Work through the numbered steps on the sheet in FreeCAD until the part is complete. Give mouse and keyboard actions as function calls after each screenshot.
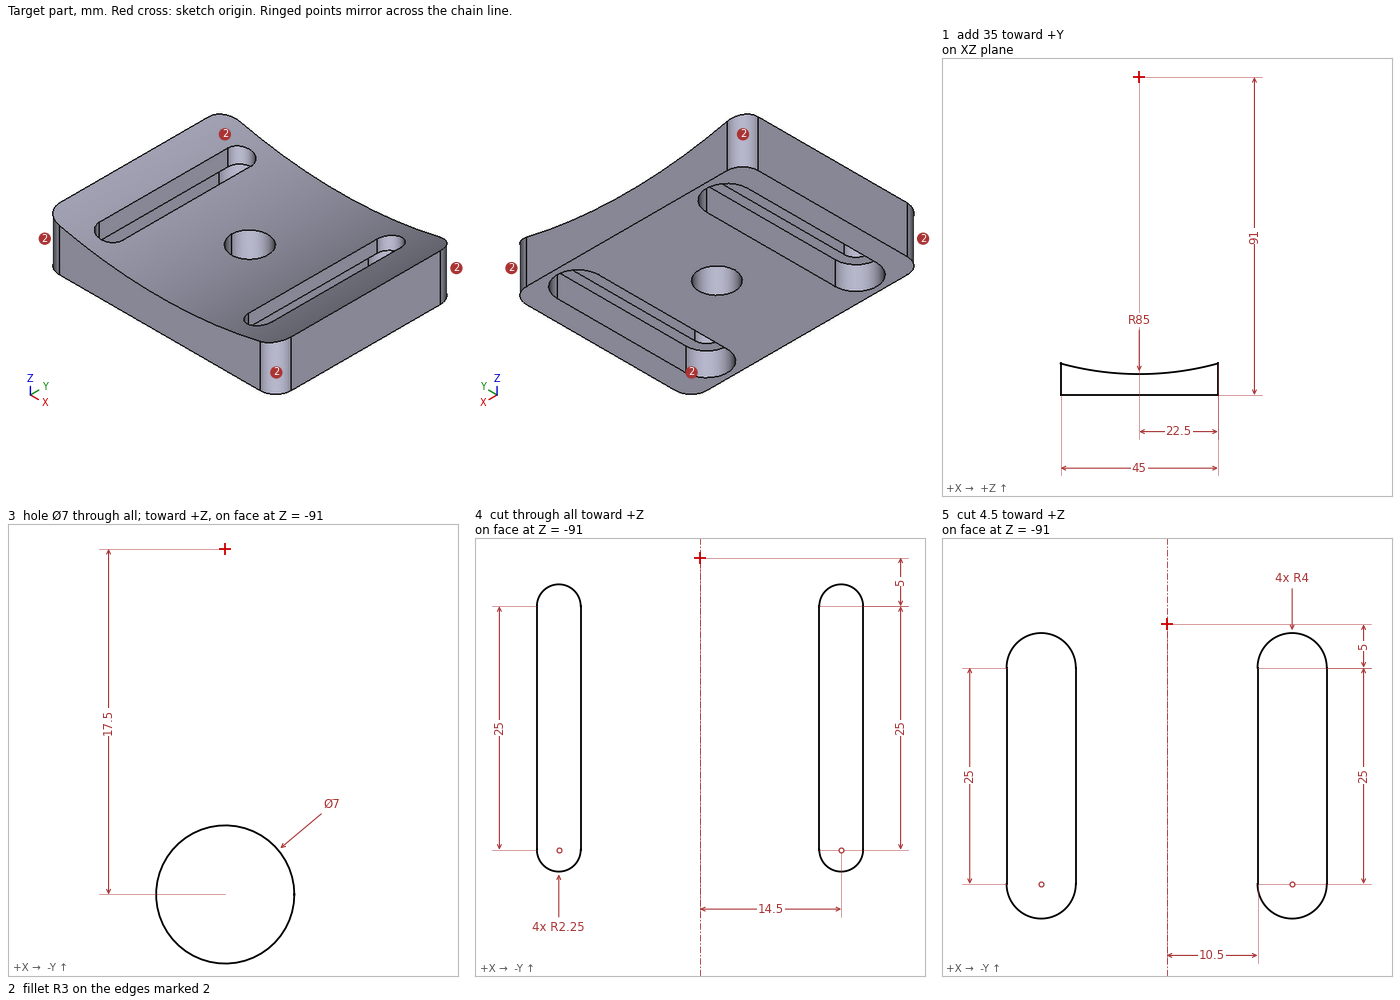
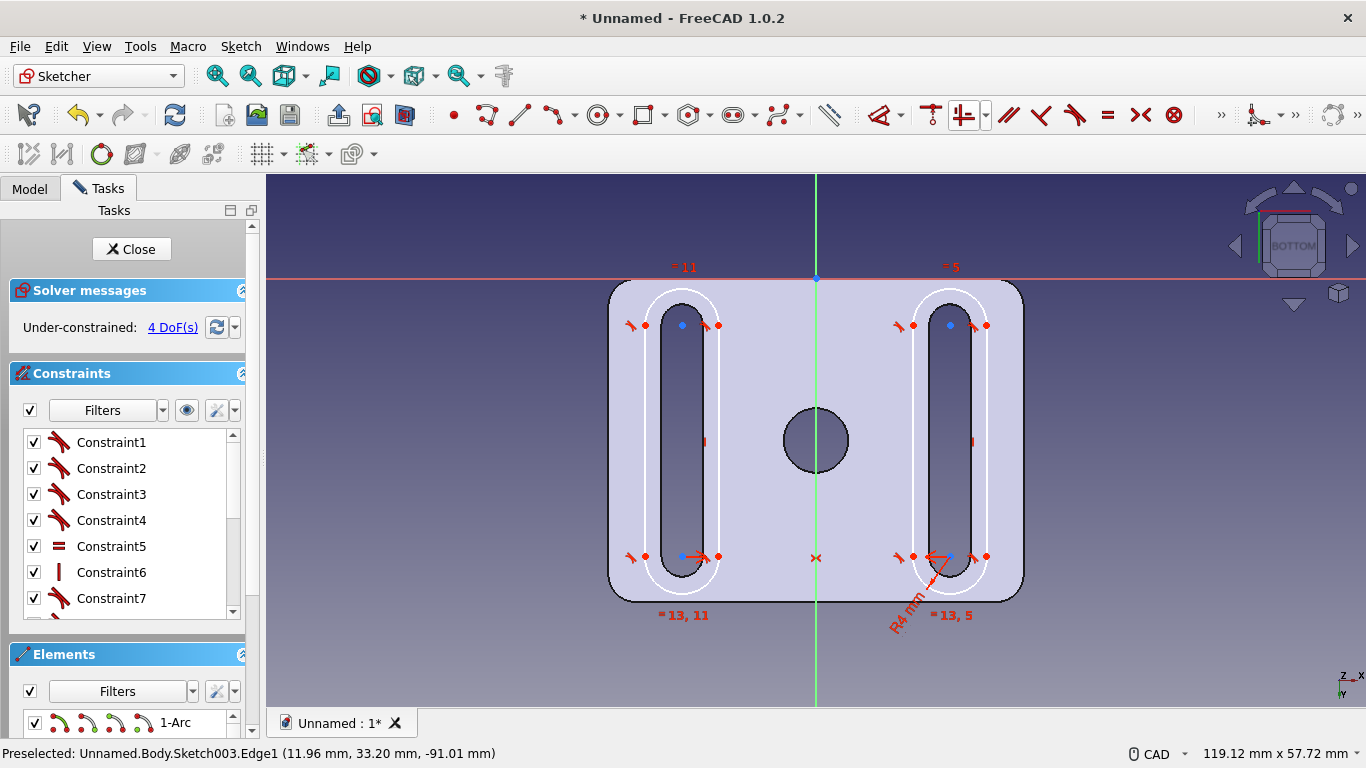
click(913, 488)
click(947, 442)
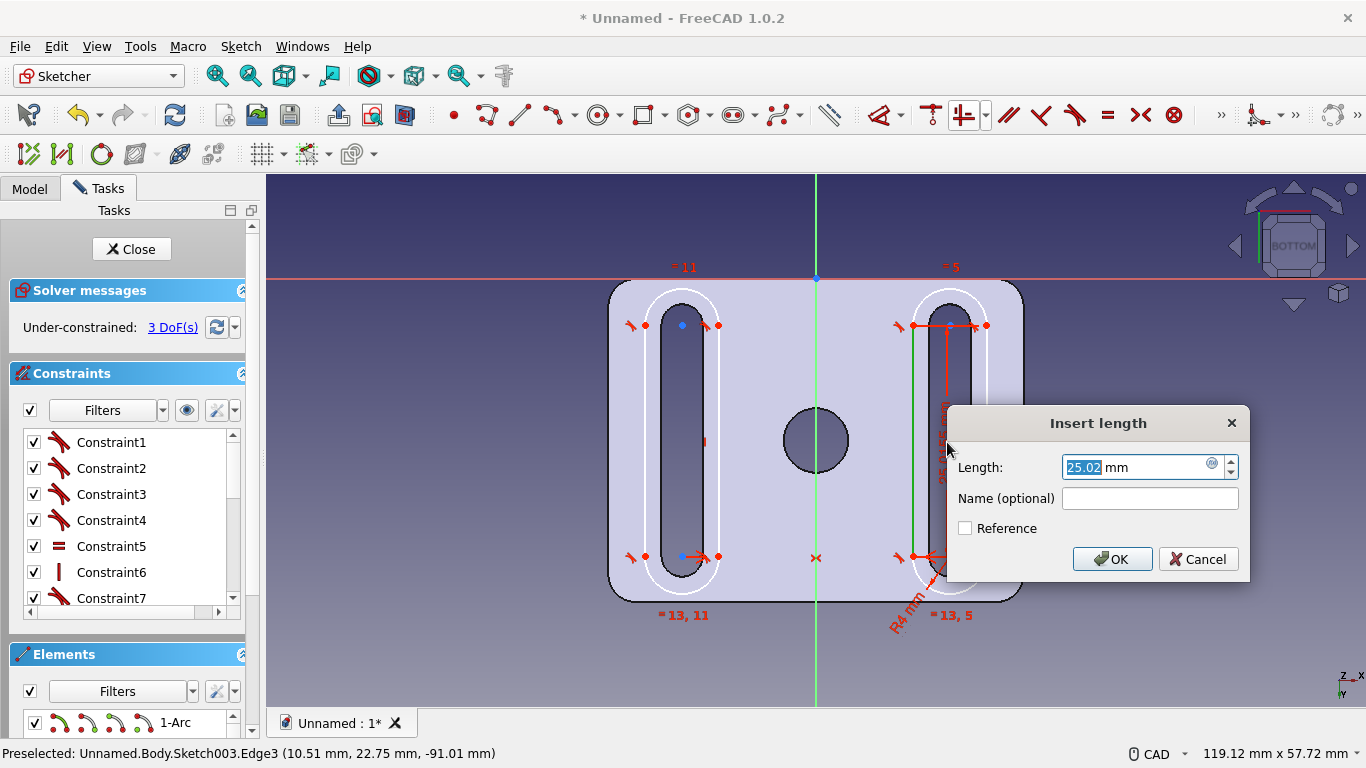
text(25)
key(Return)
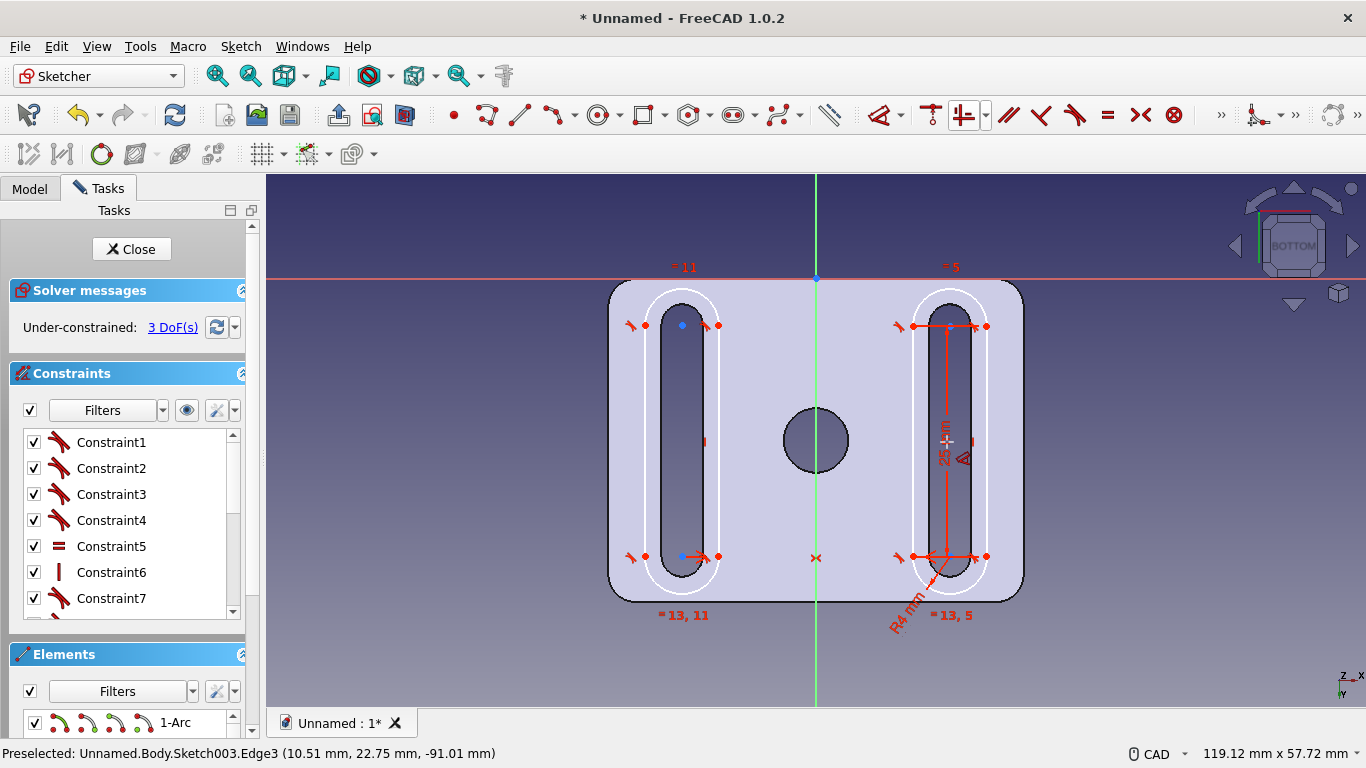
click(645, 488)
click(611, 442)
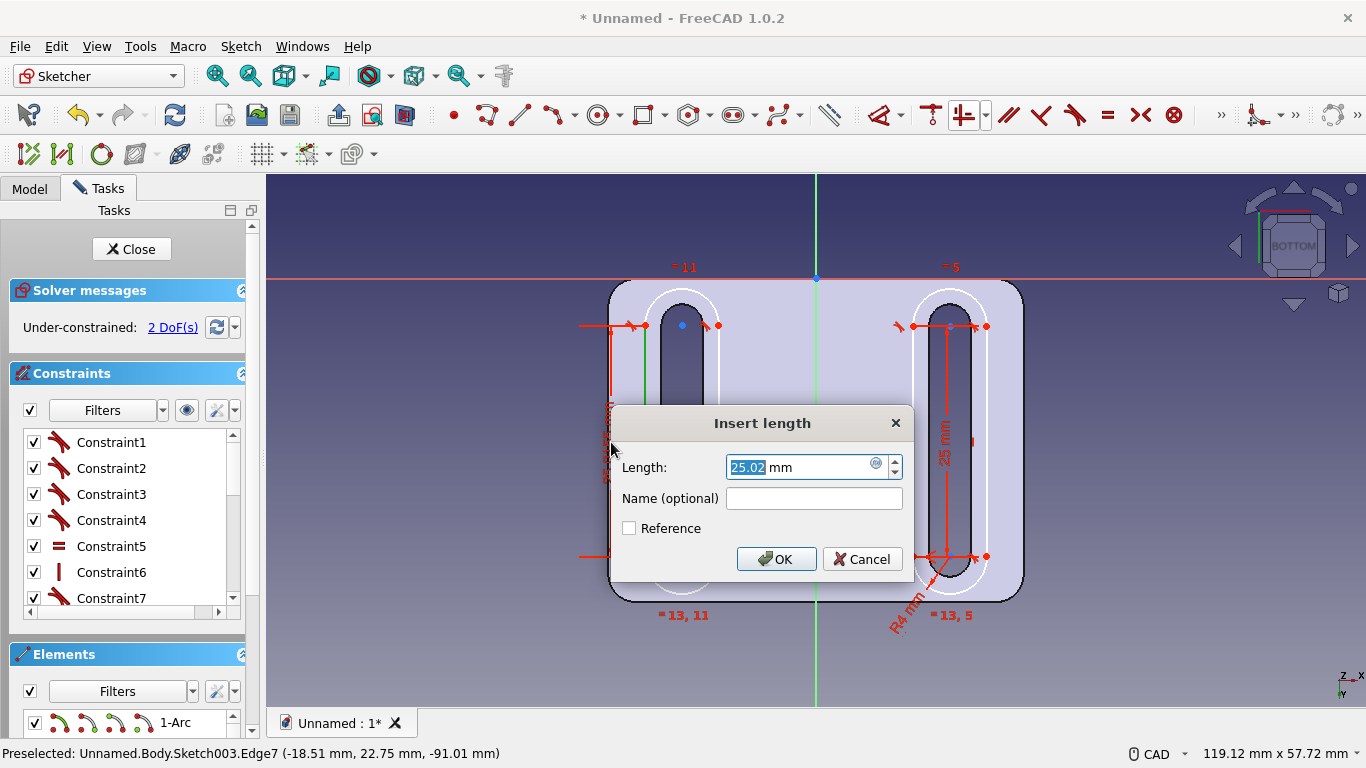
text(25)
key(Return)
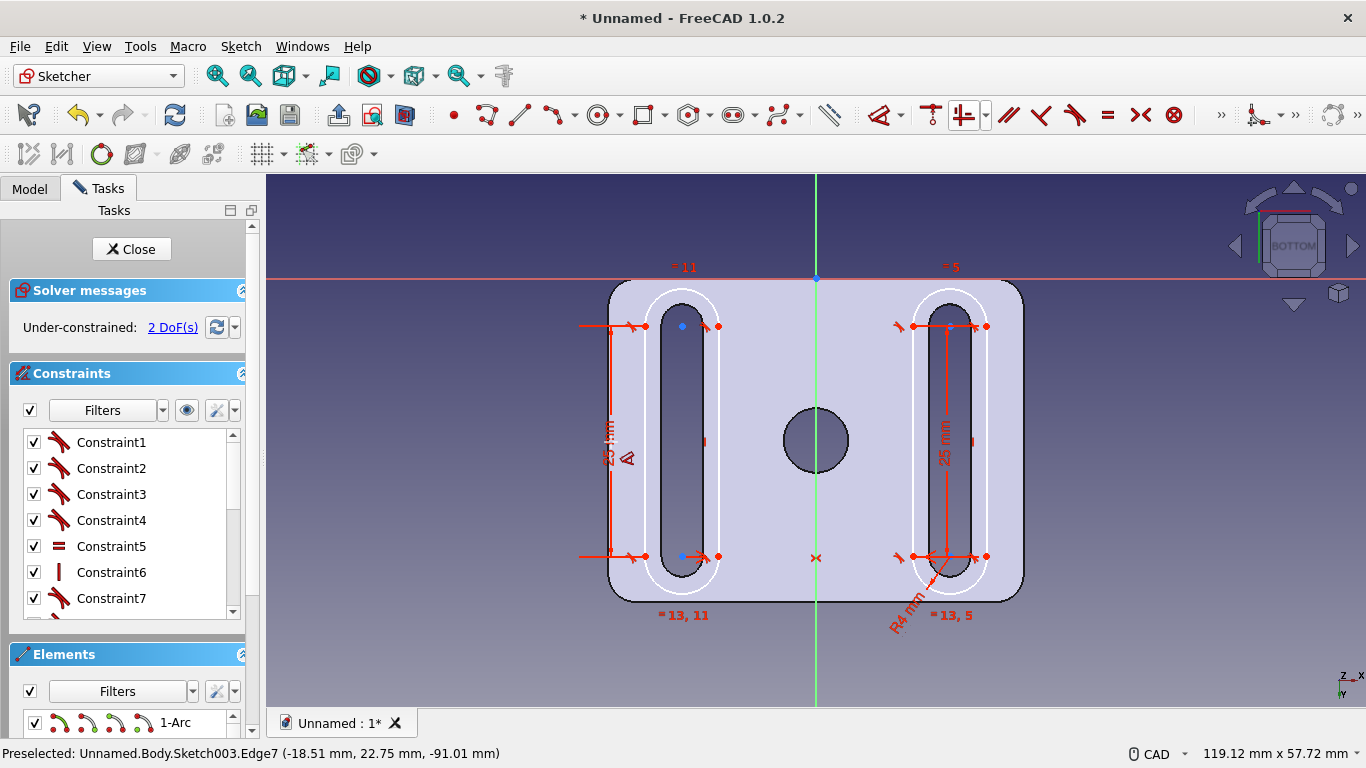
click(987, 326)
click(1021, 303)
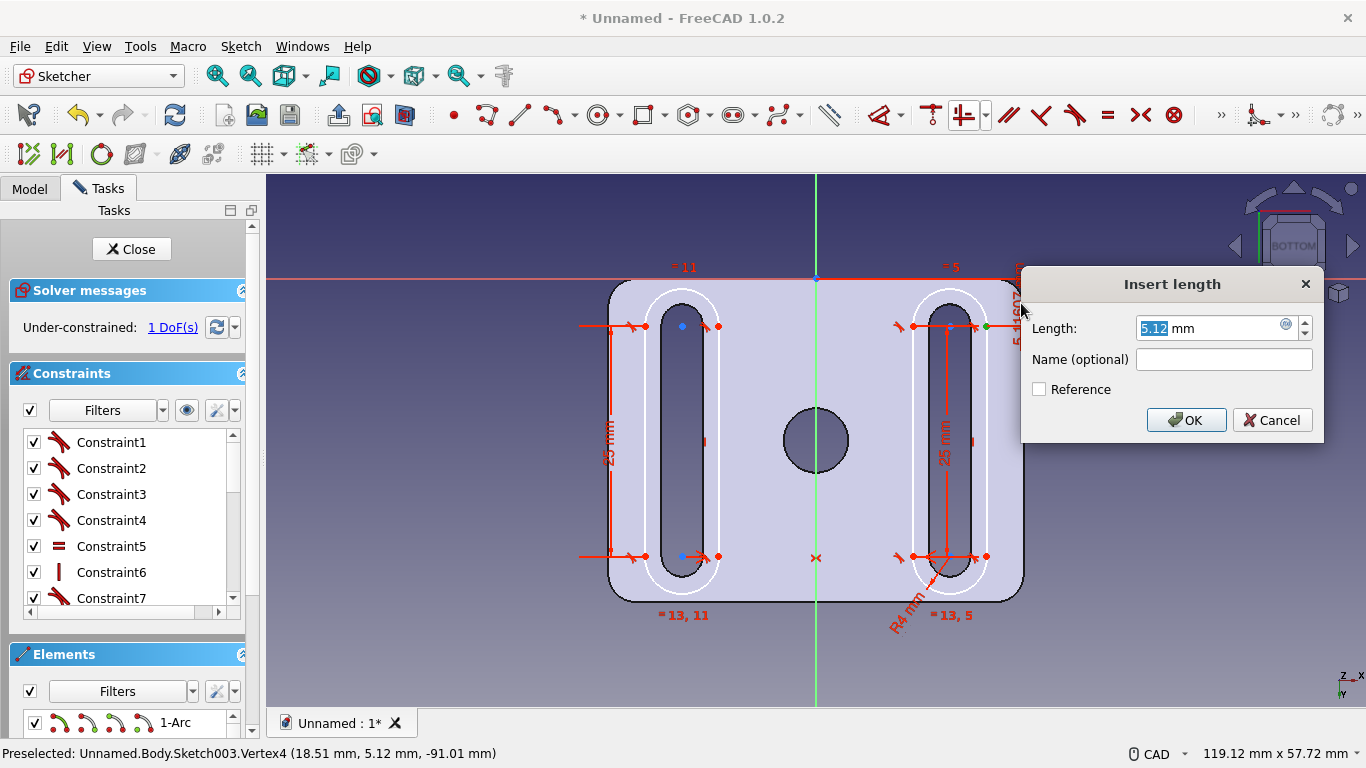
text(5)
key(Return)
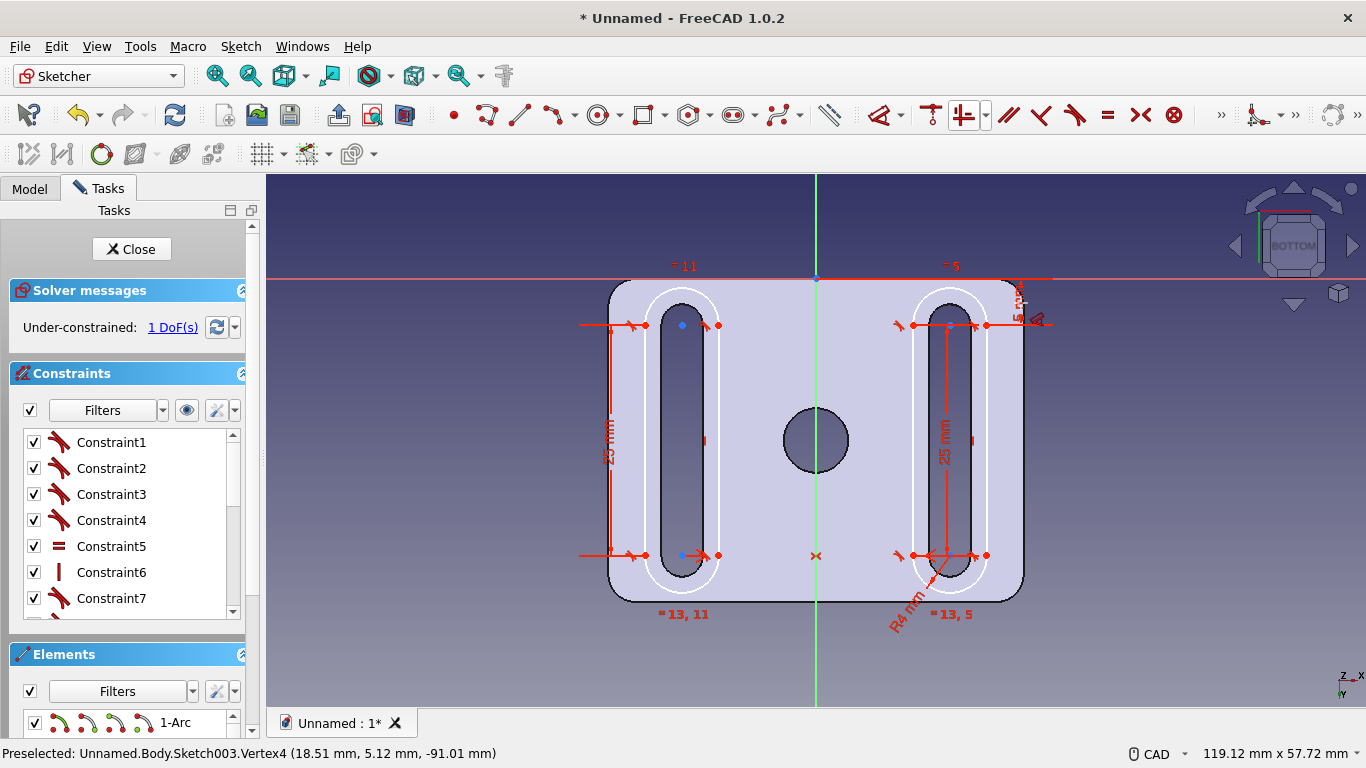
click(913, 556)
click(865, 245)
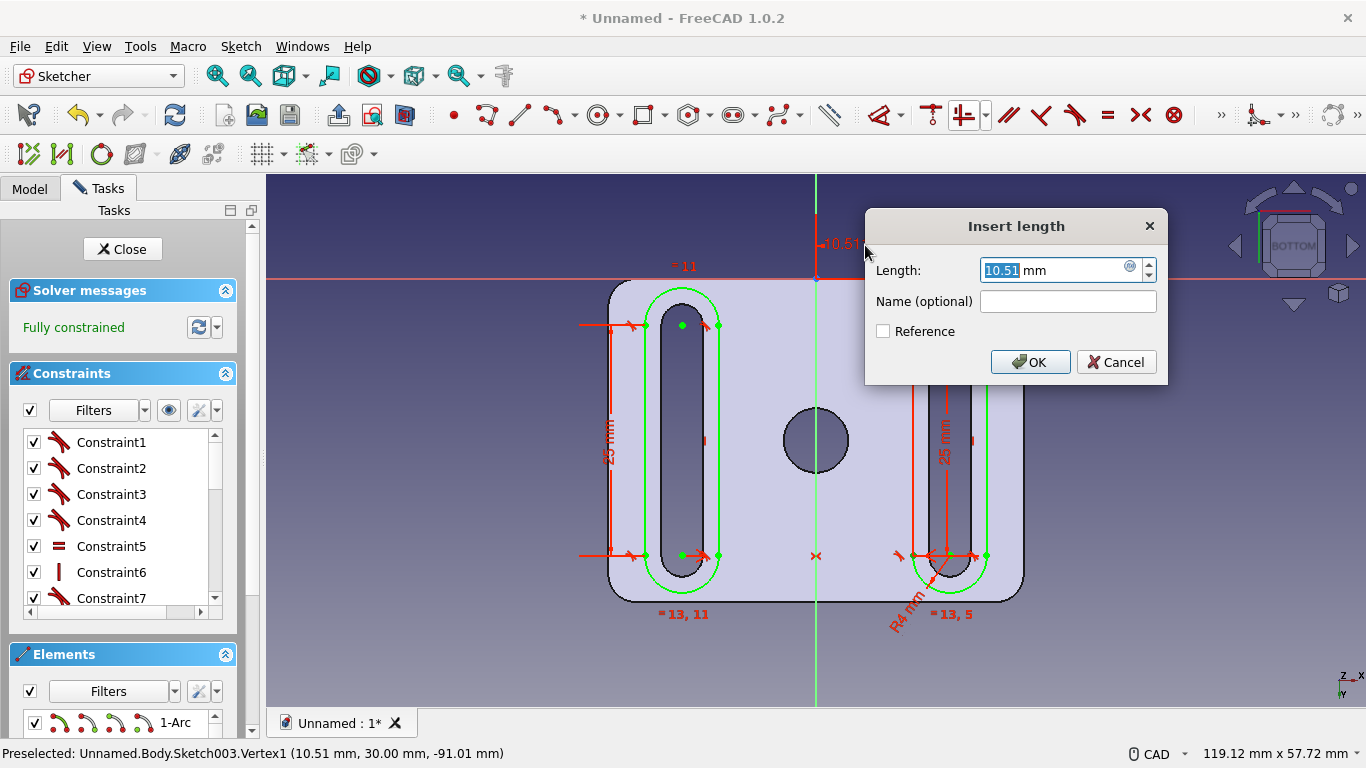
text(10.5)
key(Return)
key(Escape)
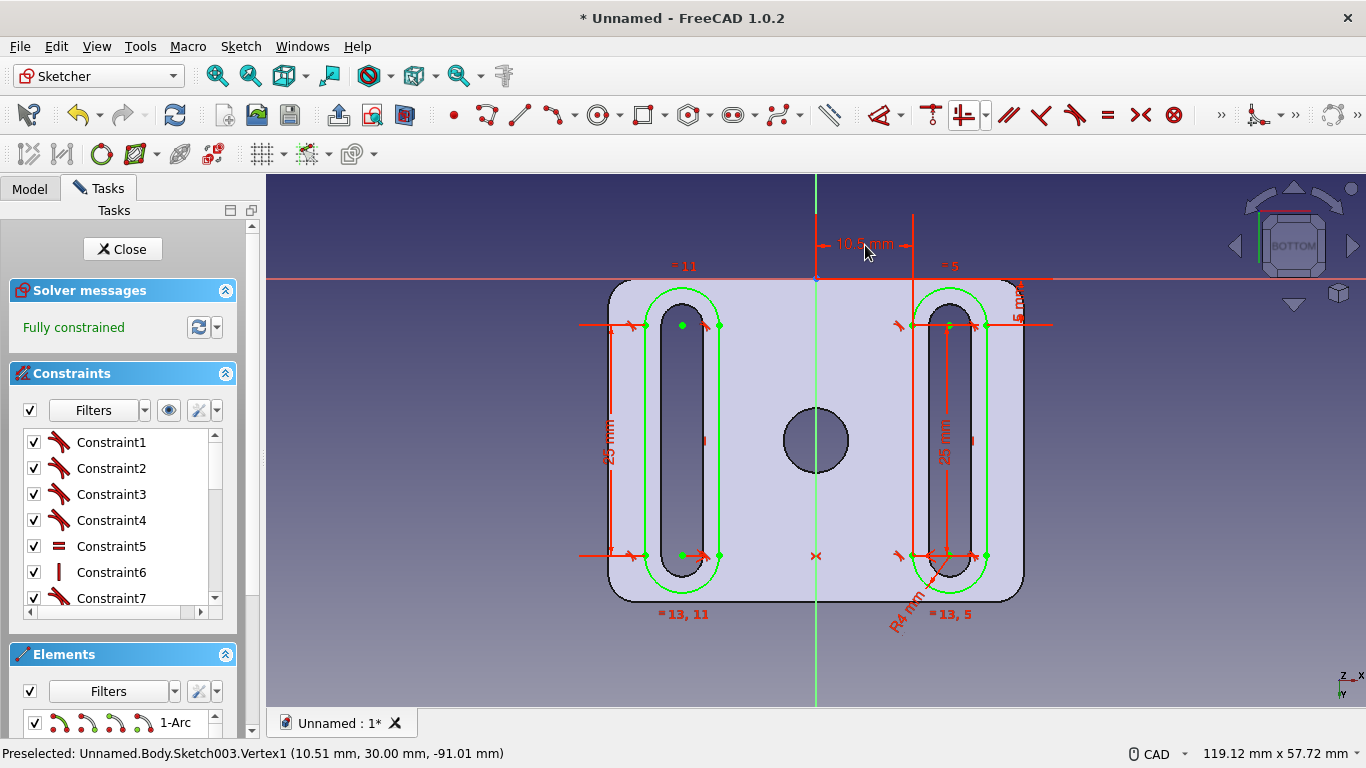
click(123, 249)